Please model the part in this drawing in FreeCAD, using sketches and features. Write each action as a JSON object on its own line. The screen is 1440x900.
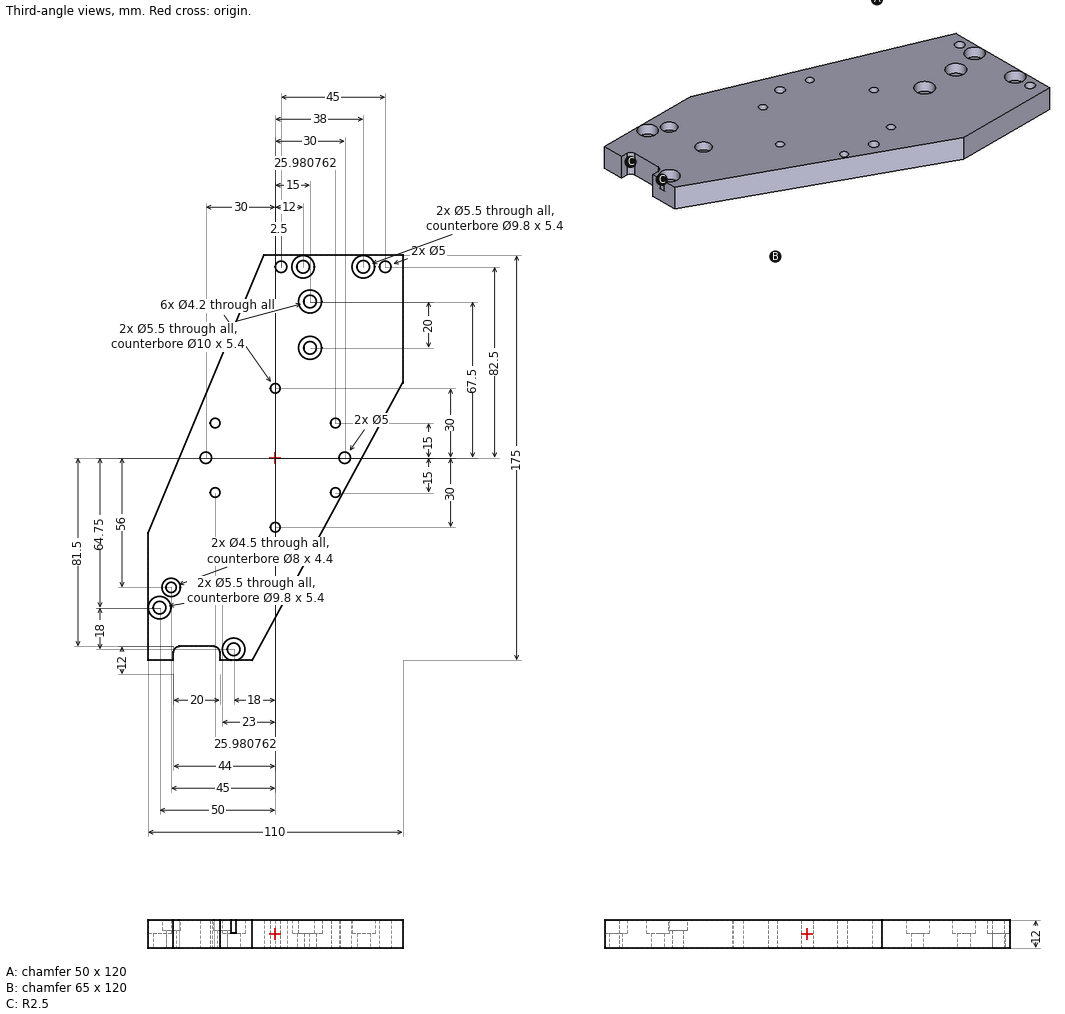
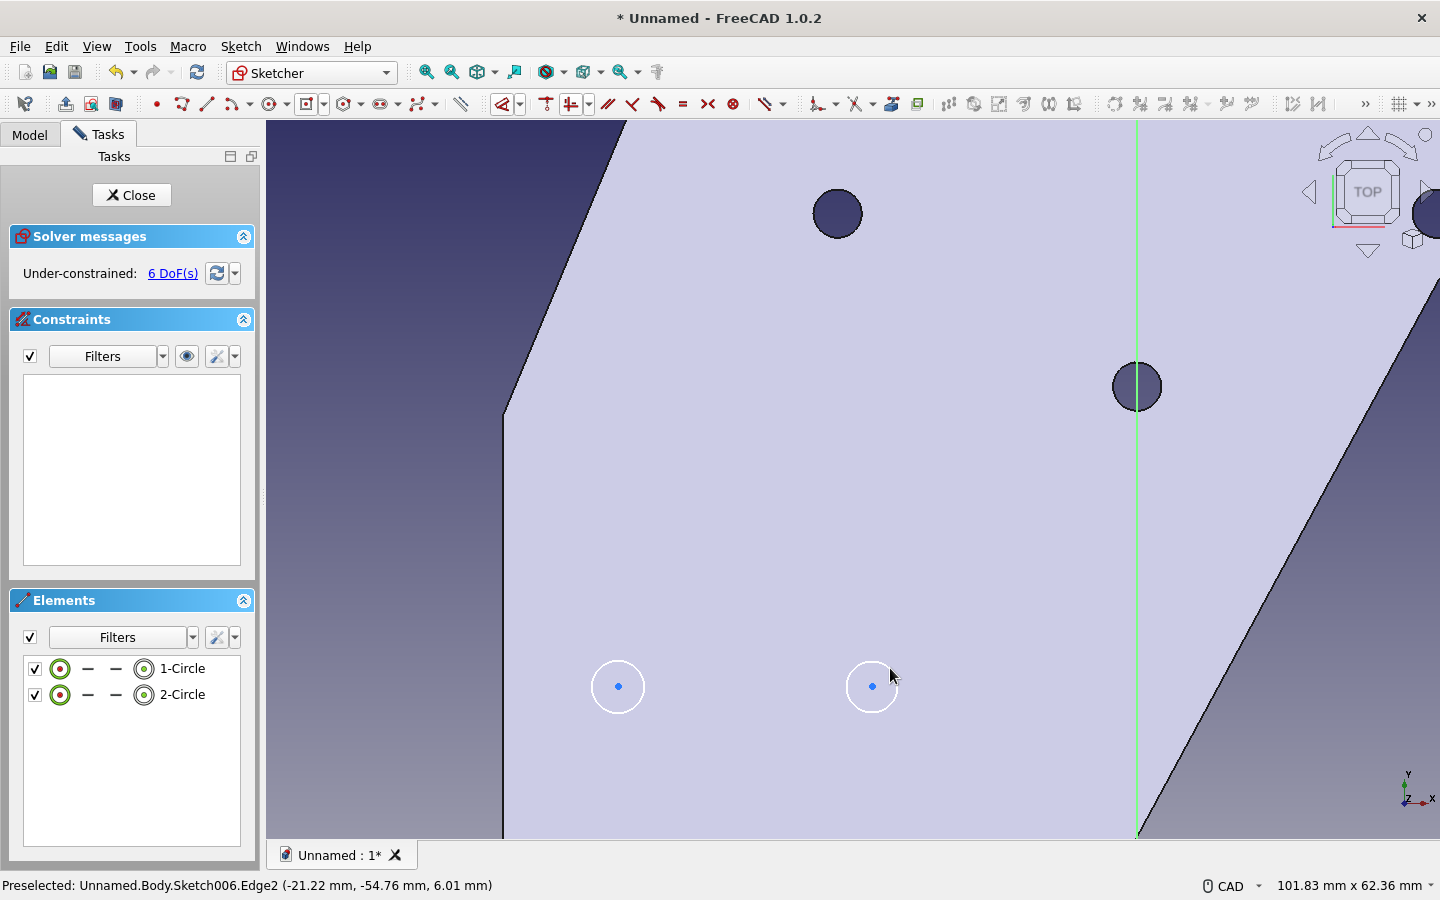
{"action": "left_click", "coordinate": [636, 668]}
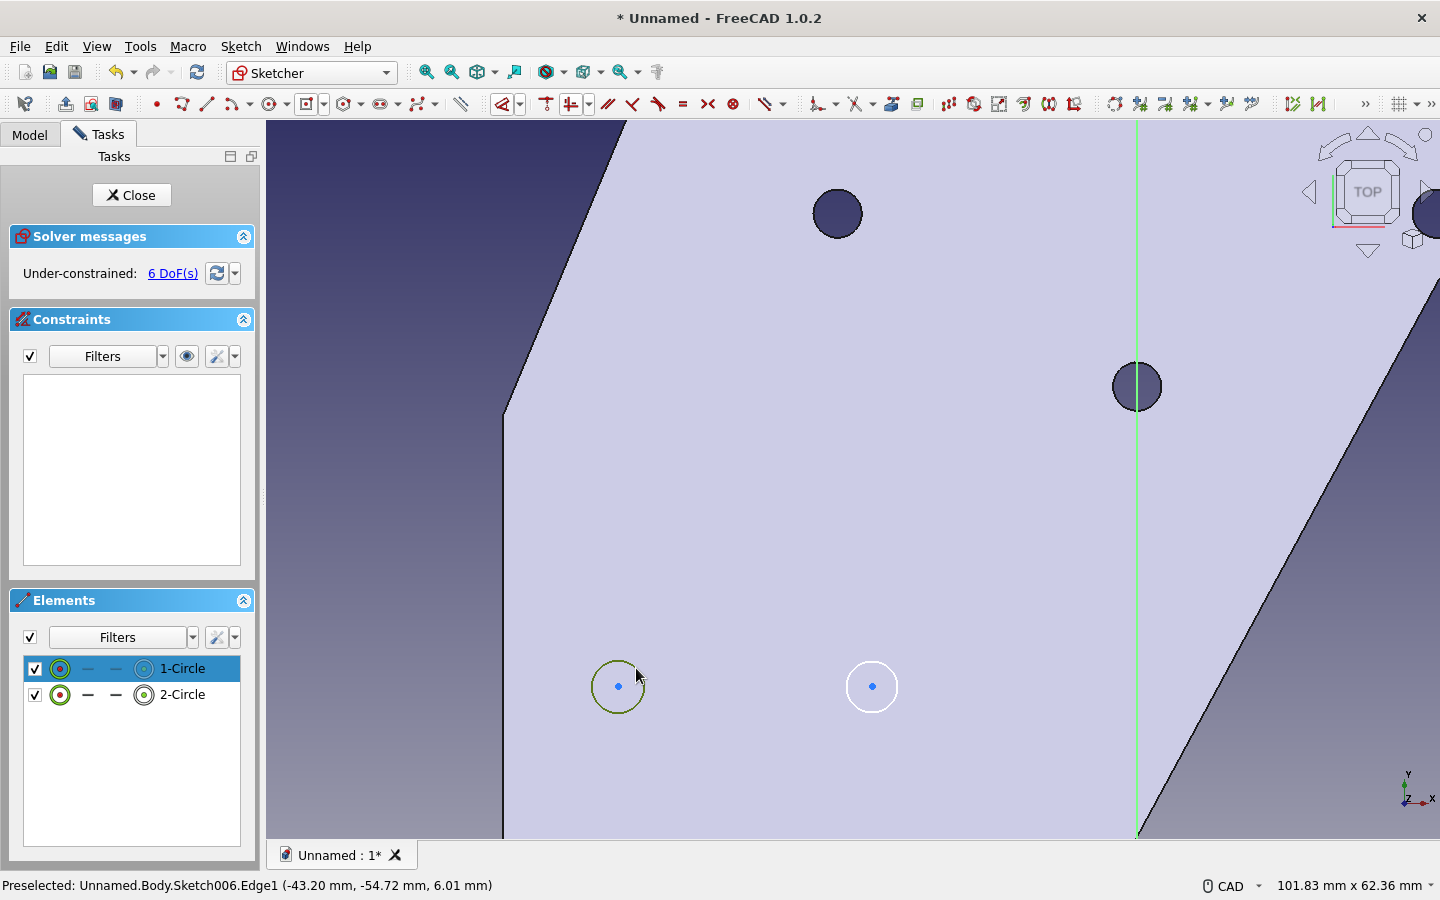
{"action": "left_click", "coordinate": [890, 669]}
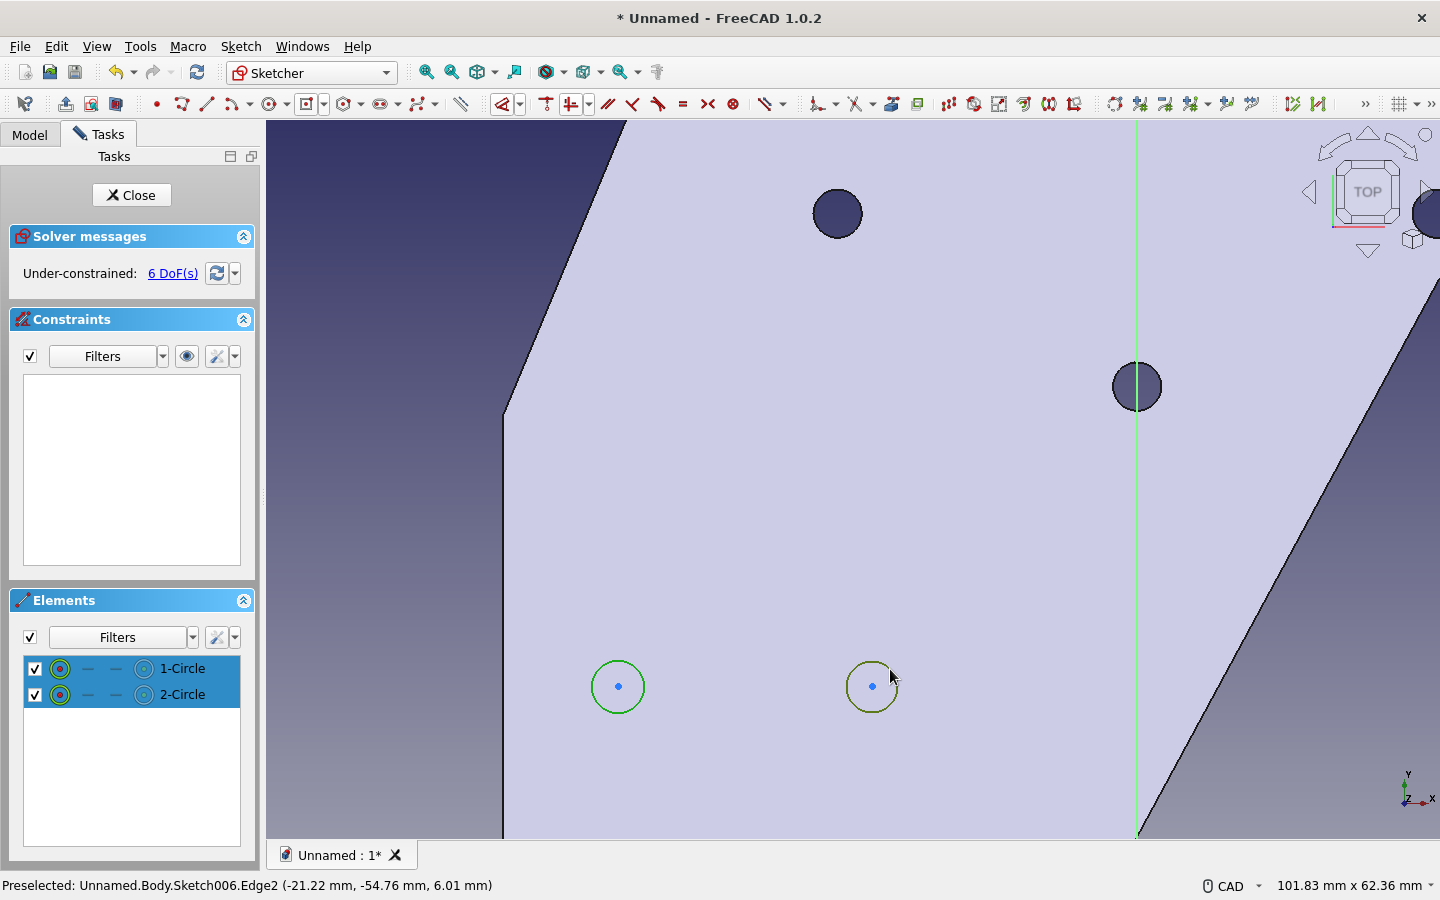
{"action": "key", "text": "e"}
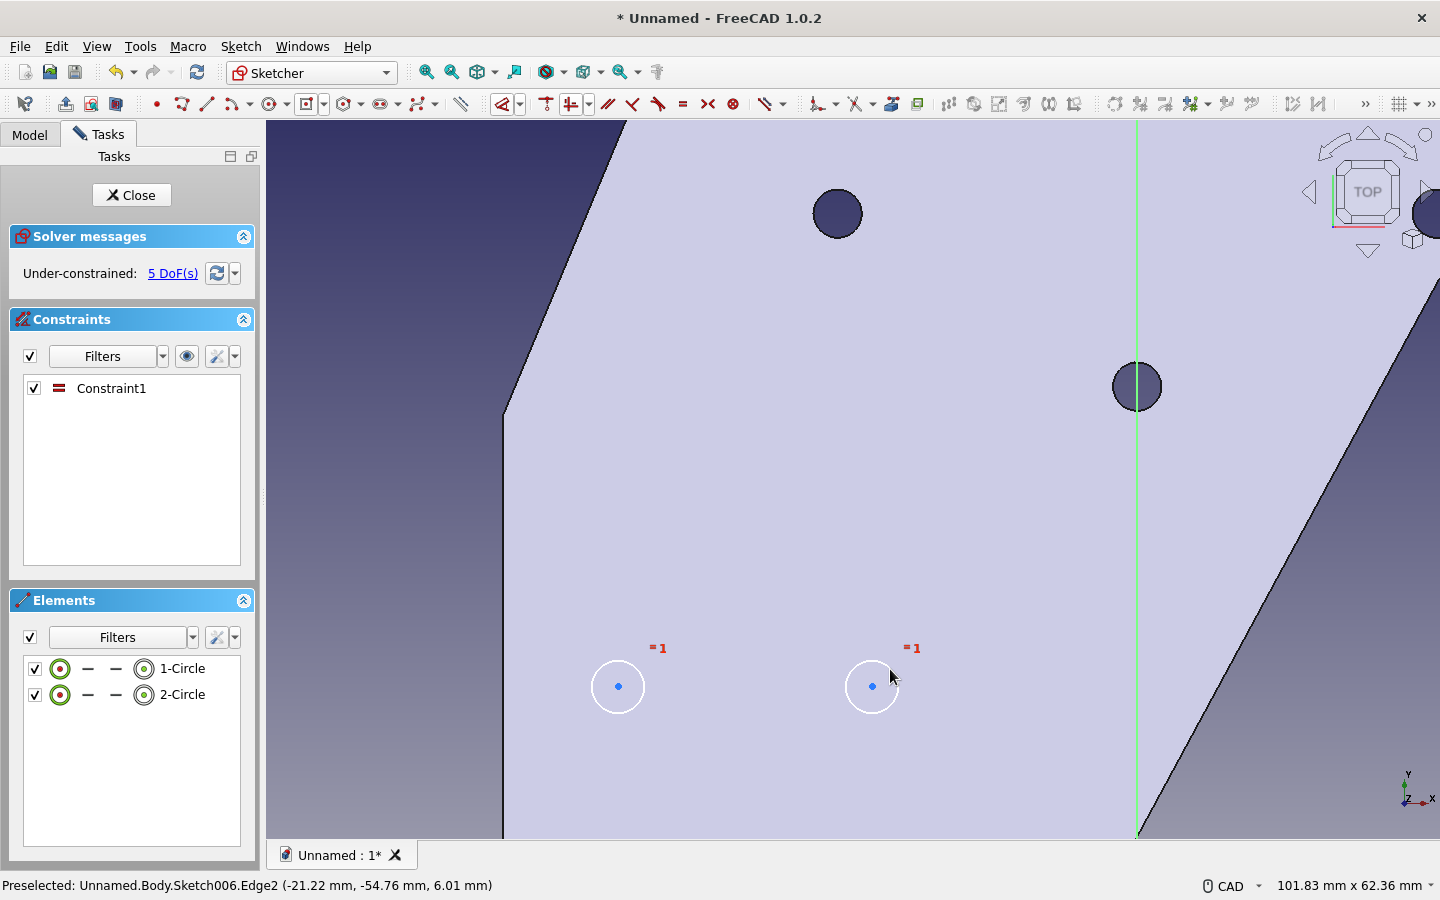
{"action": "left_click", "coordinate": [618, 687]}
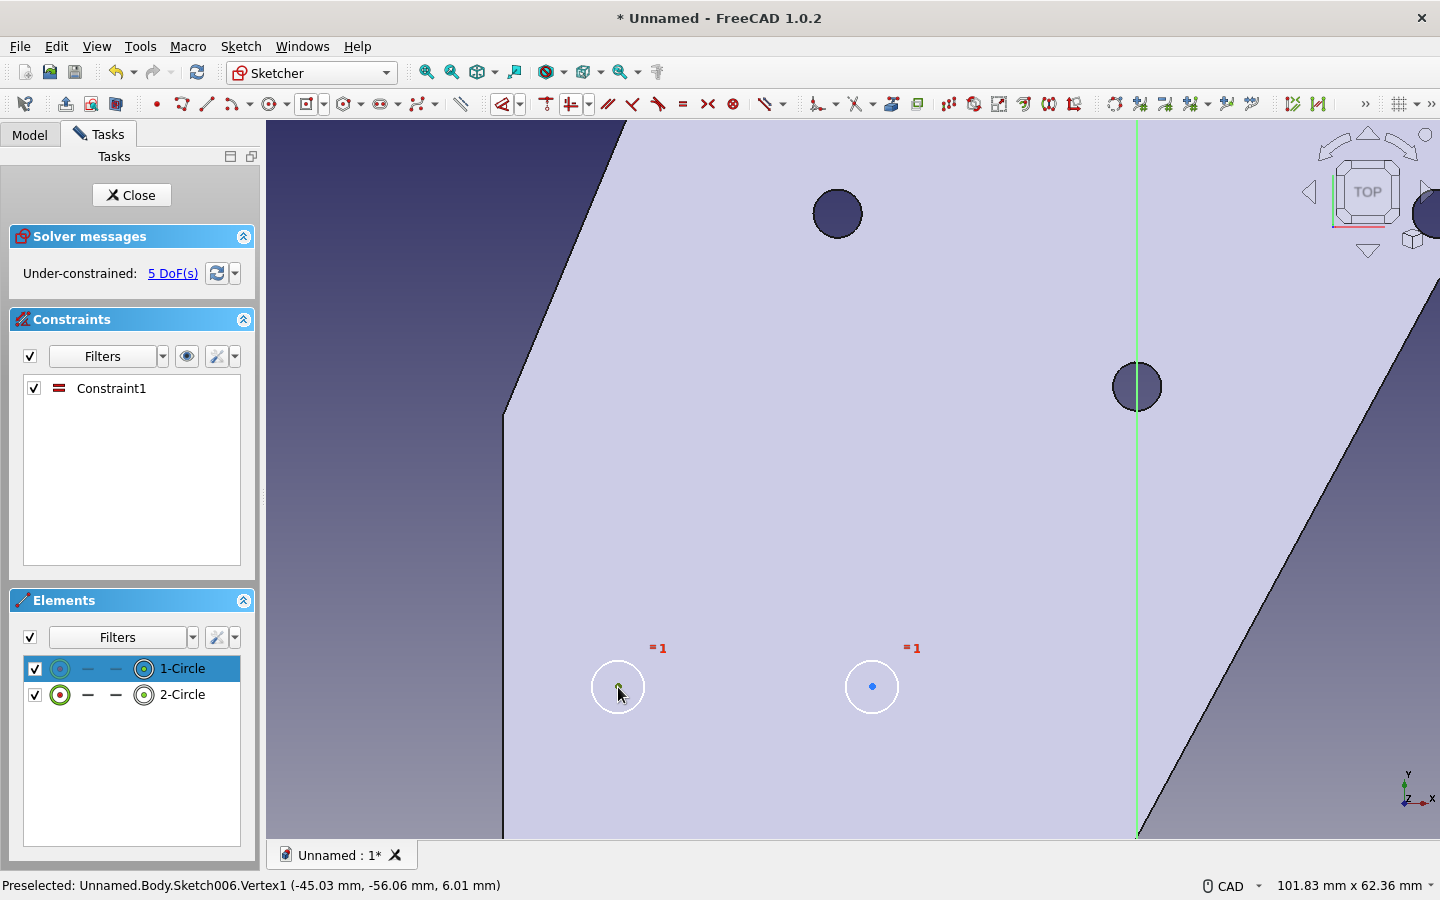
{"action": "left_click", "coordinate": [872, 687]}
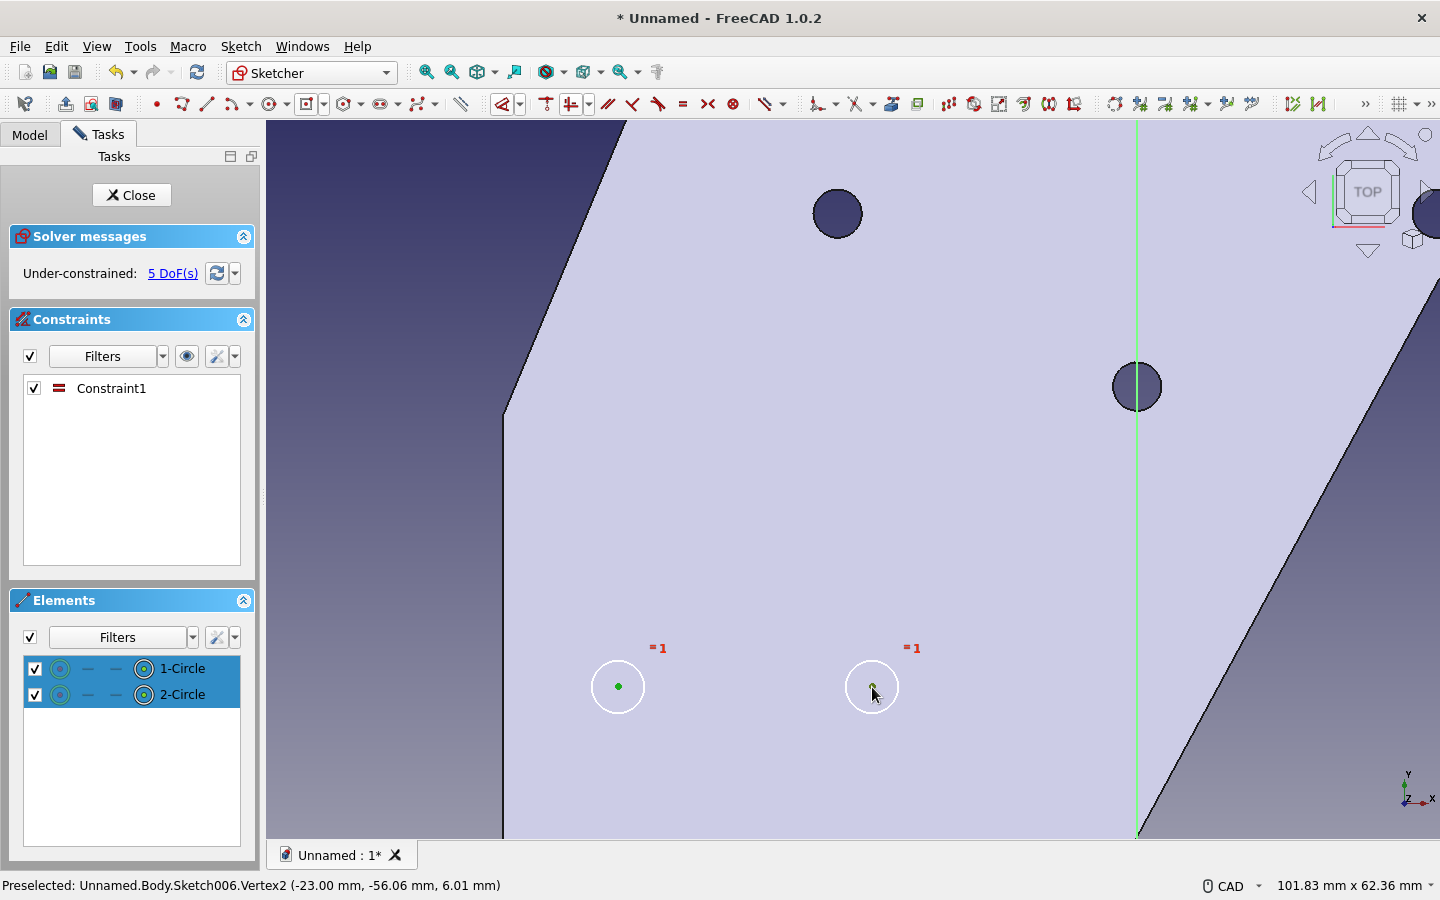
{"action": "key", "text": "h"}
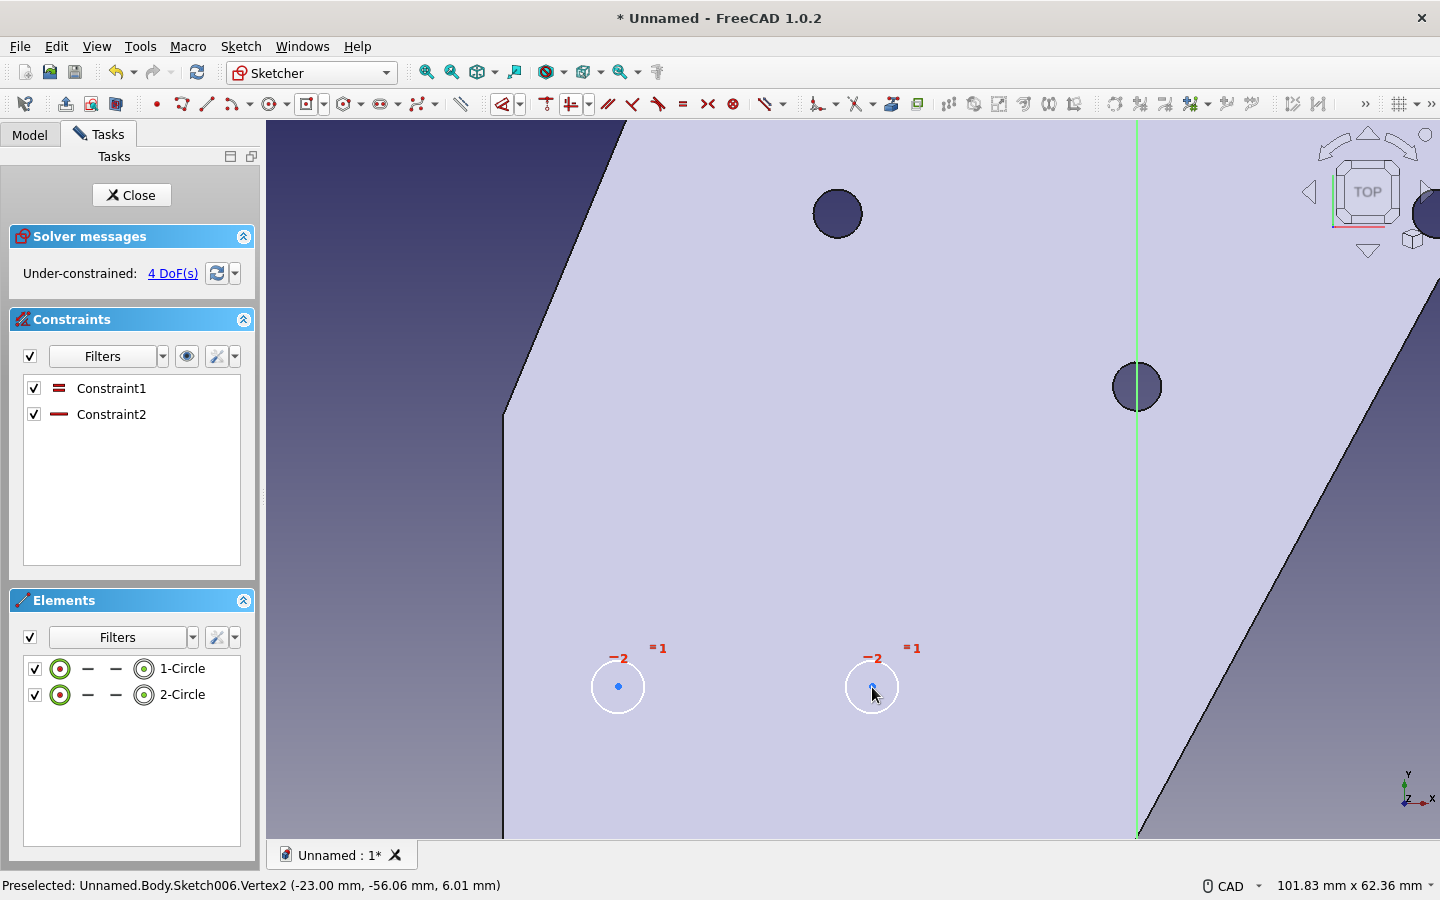
{"action": "left_click", "coordinate": [636, 668]}